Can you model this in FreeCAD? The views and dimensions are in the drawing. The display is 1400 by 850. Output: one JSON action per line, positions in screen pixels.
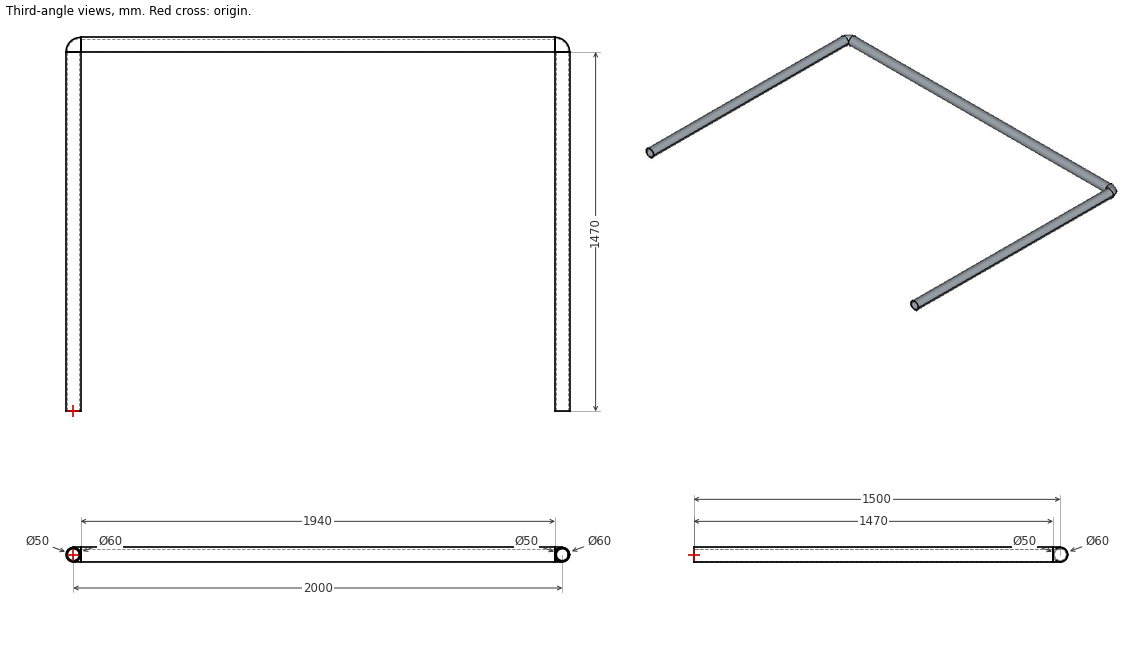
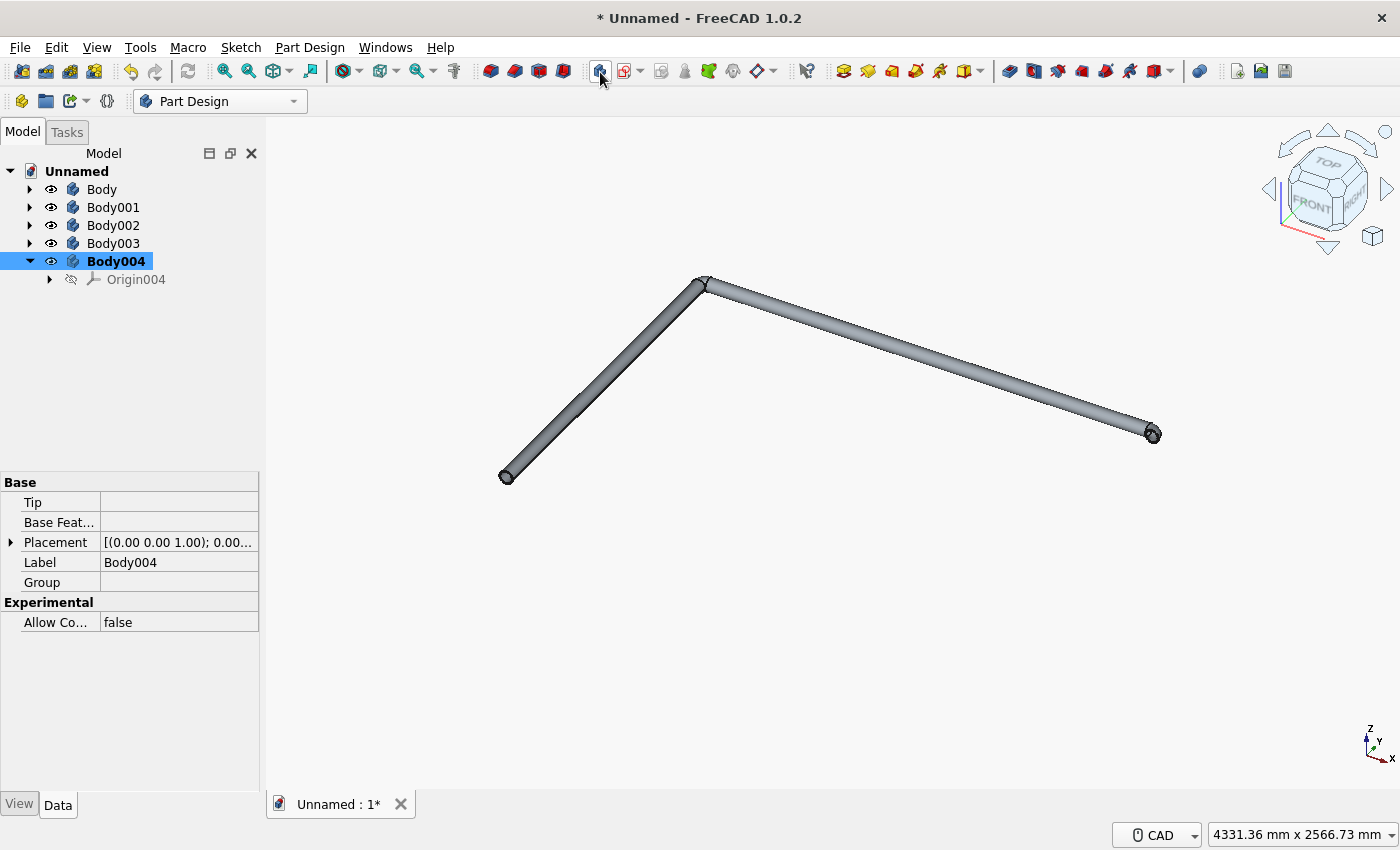
{"action": "left_click", "coordinate": [306, 749]}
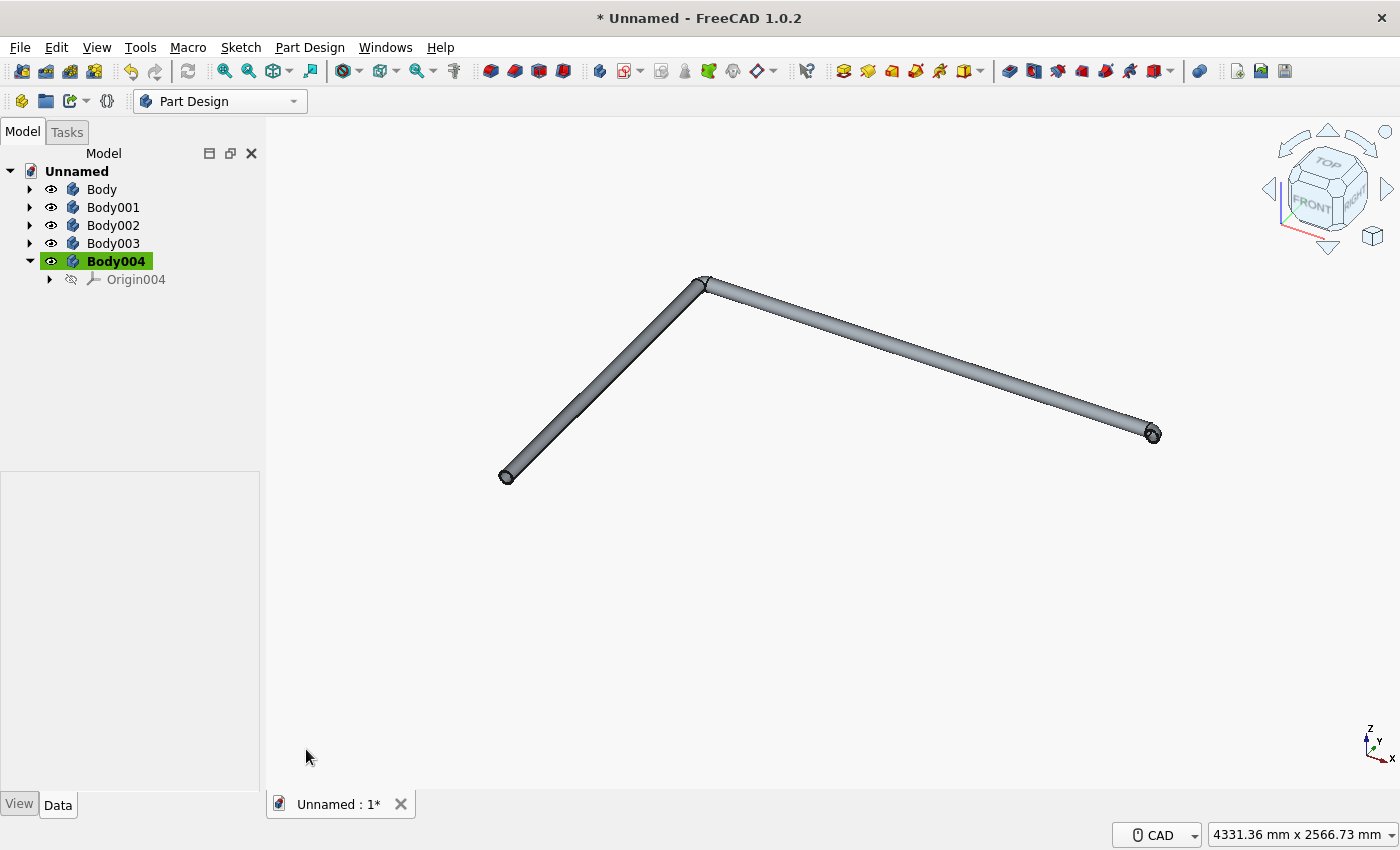
{"action": "left_click", "coordinate": [624, 72]}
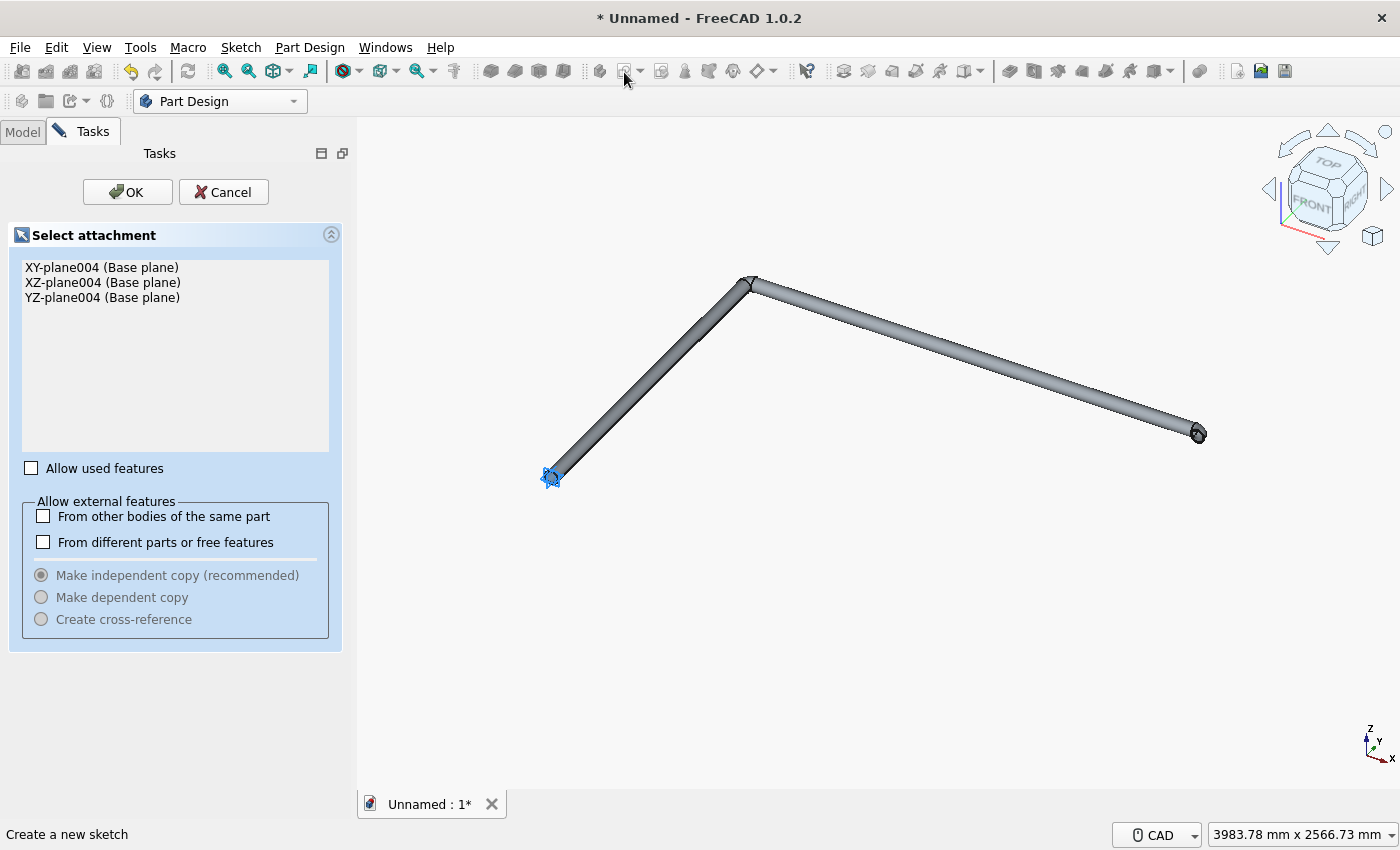
{"action": "left_click", "coordinate": [82, 282]}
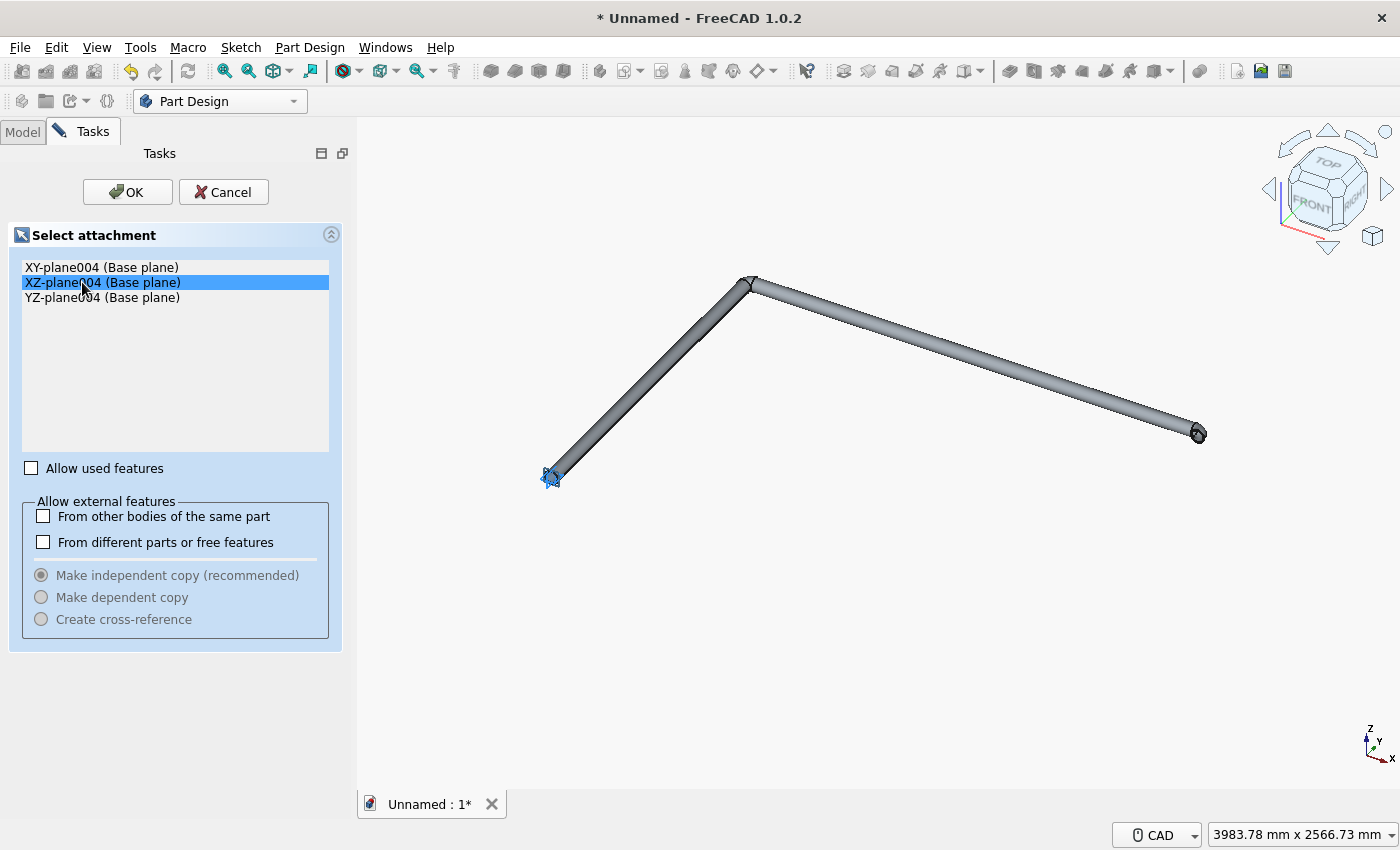
{"action": "left_click", "coordinate": [128, 192]}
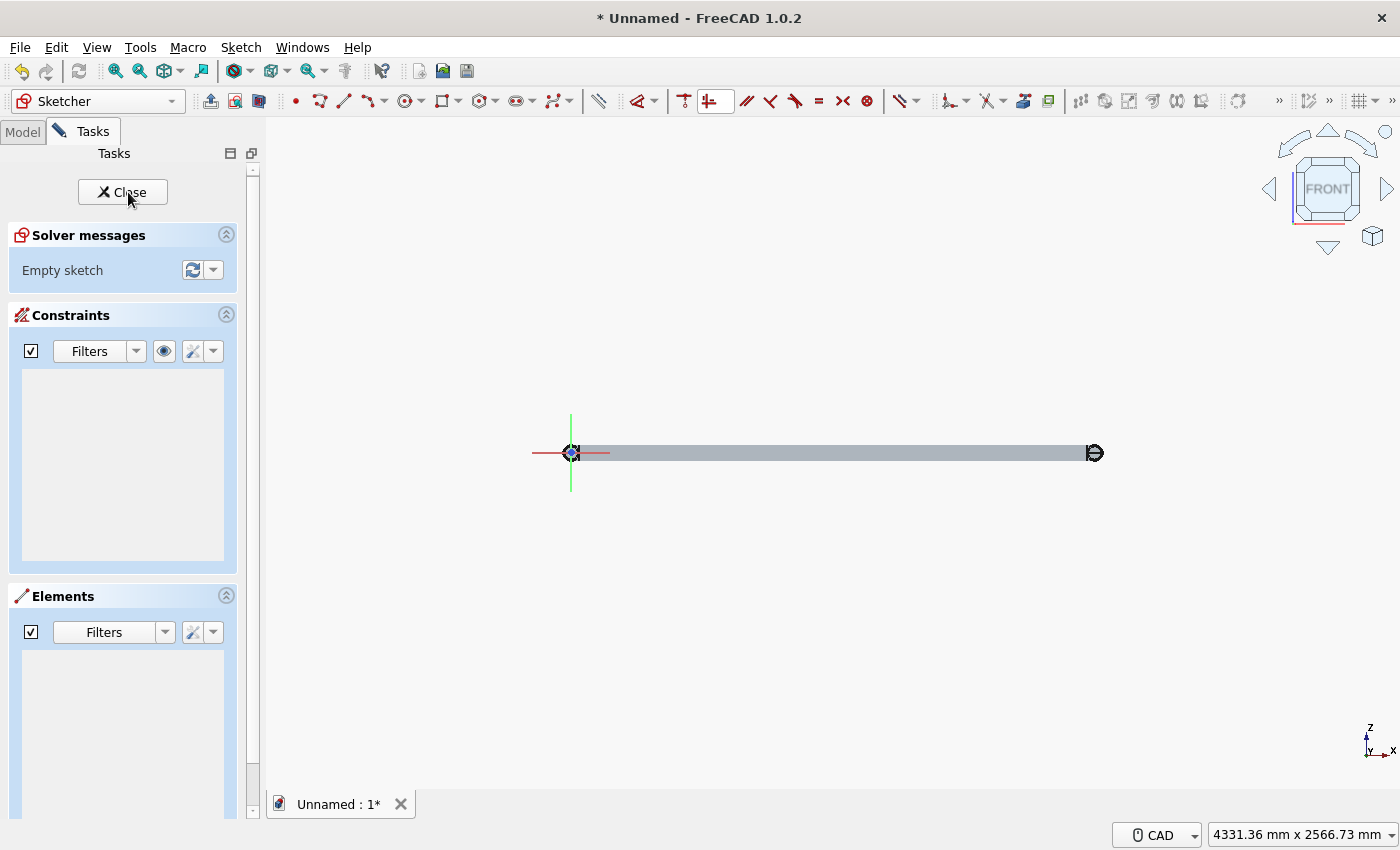
{"action": "scroll", "coordinate": [1112, 453], "scroll_direction": "up", "scroll_amount": 15}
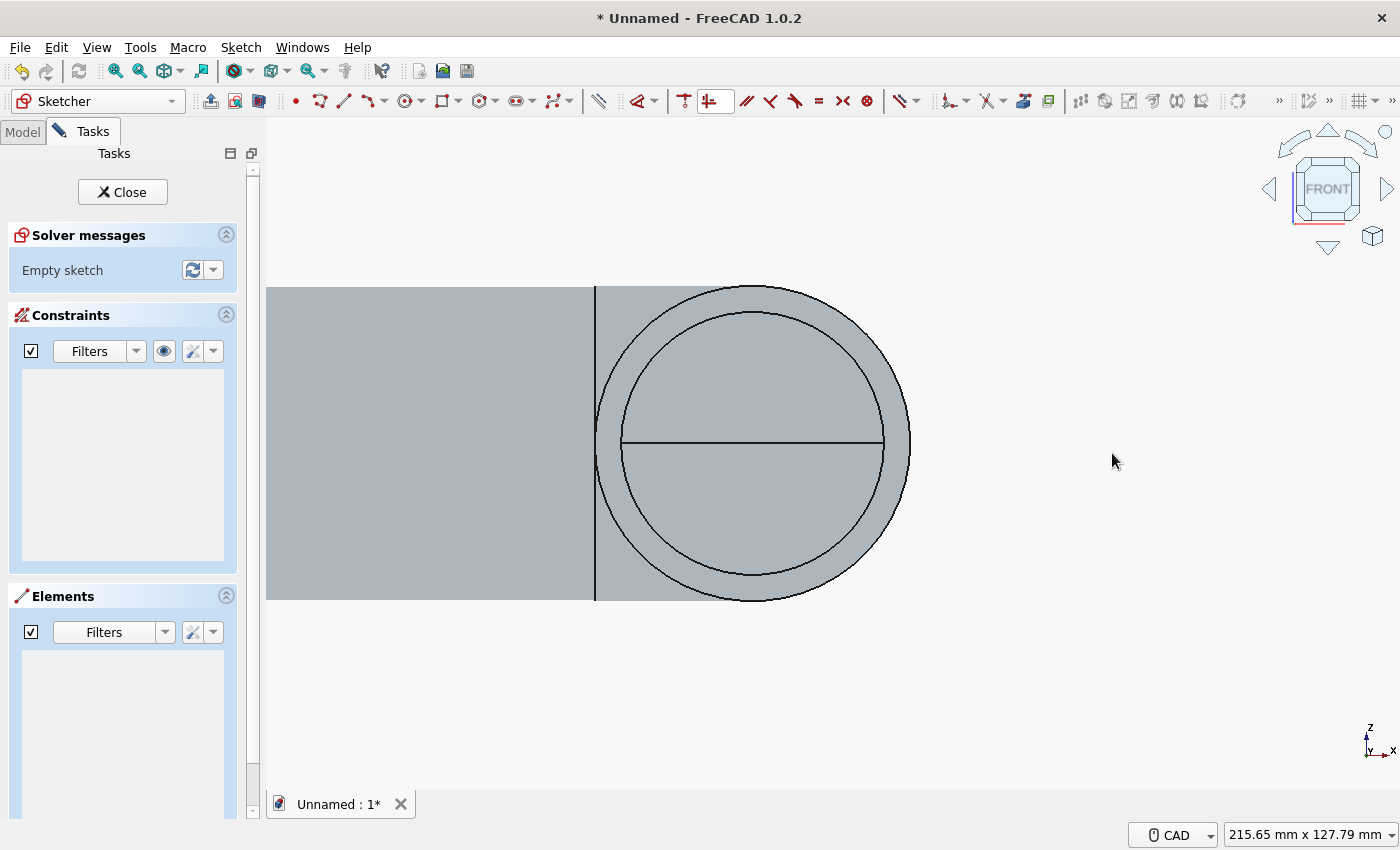
{"action": "scroll", "coordinate": [728, 424], "scroll_direction": "up", "scroll_amount": 2}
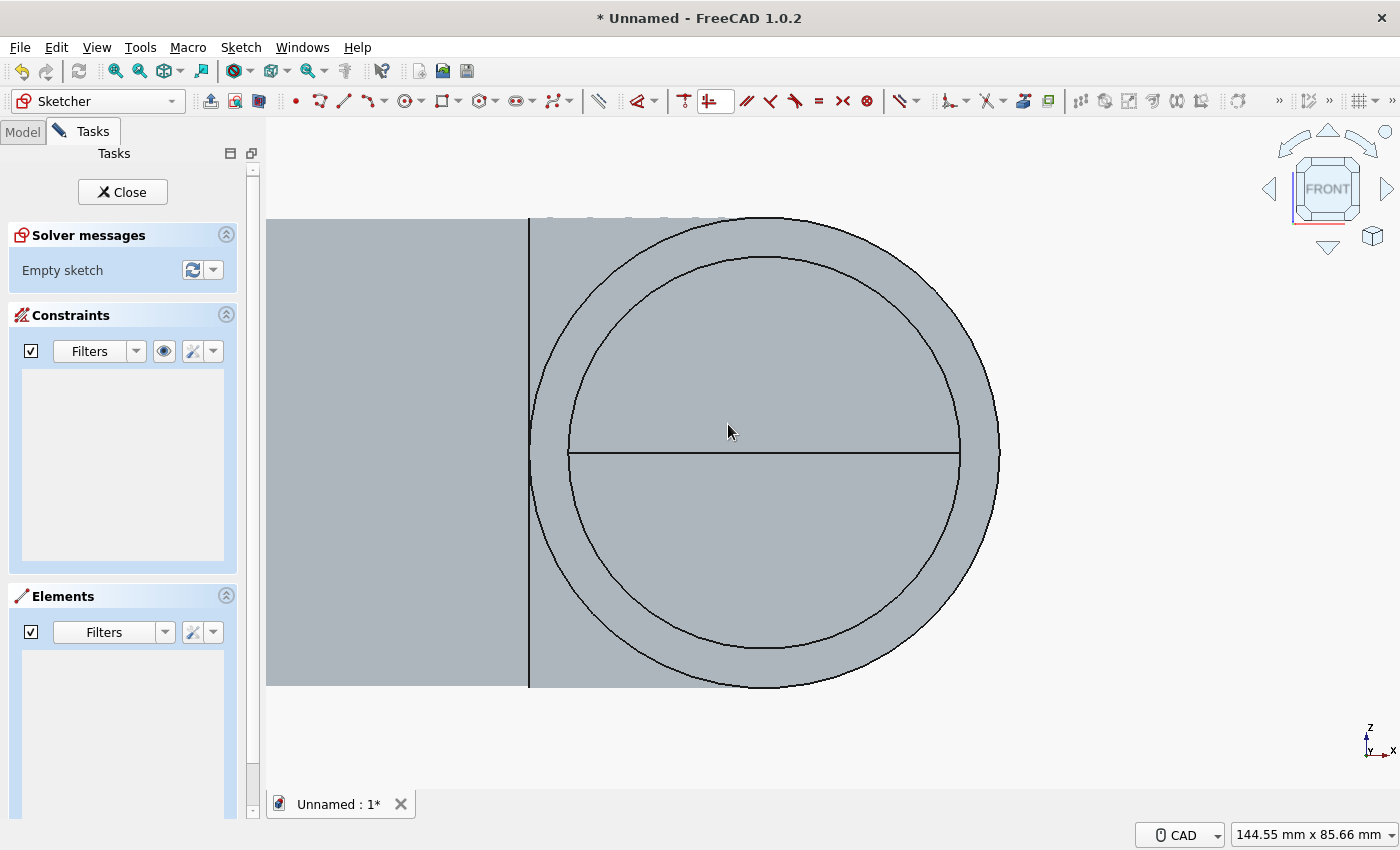
{"action": "left_click", "coordinate": [406, 102]}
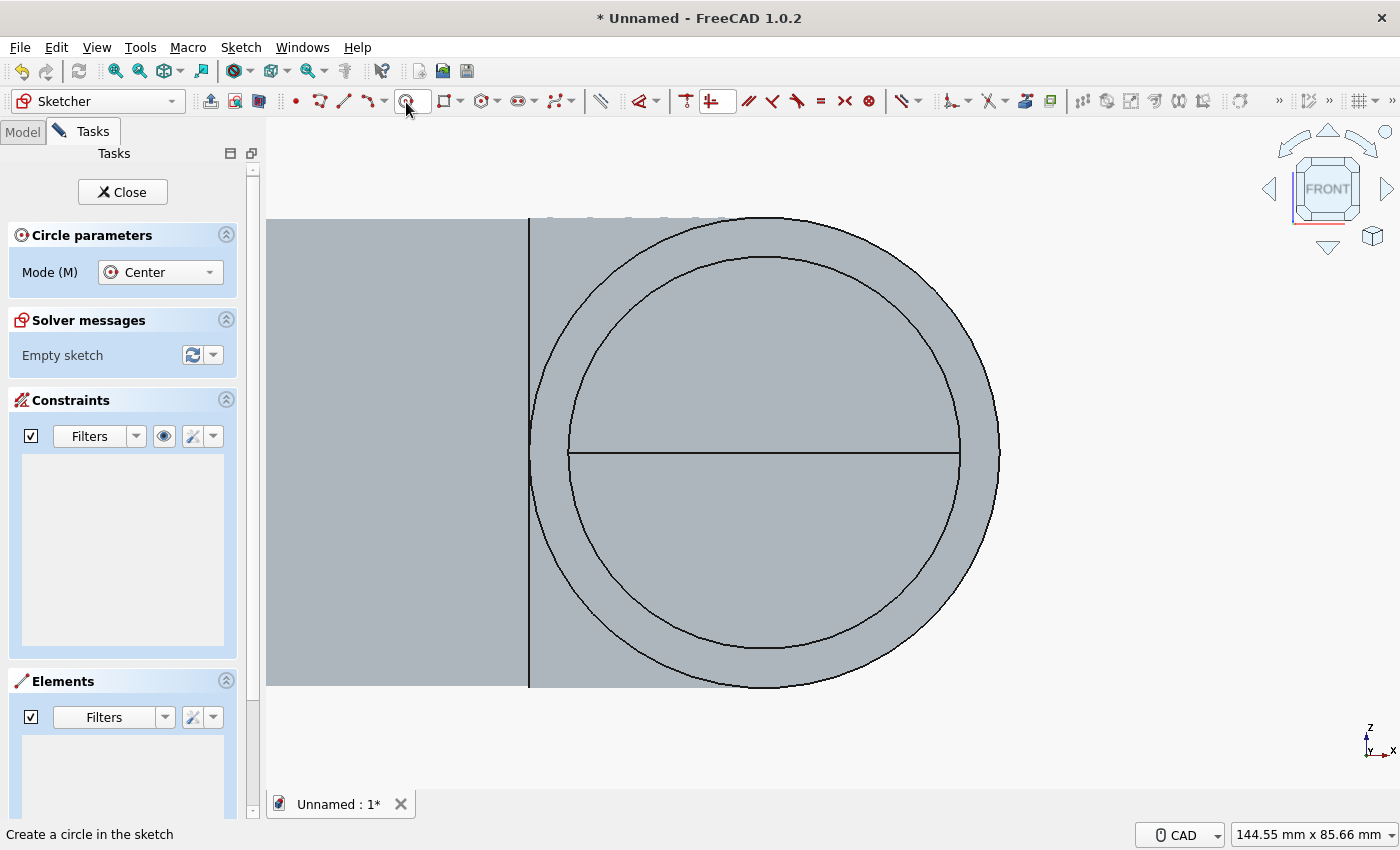
{"action": "left_click", "coordinate": [764, 453]}
{"action": "mouse_move", "coordinate": [931, 286]}